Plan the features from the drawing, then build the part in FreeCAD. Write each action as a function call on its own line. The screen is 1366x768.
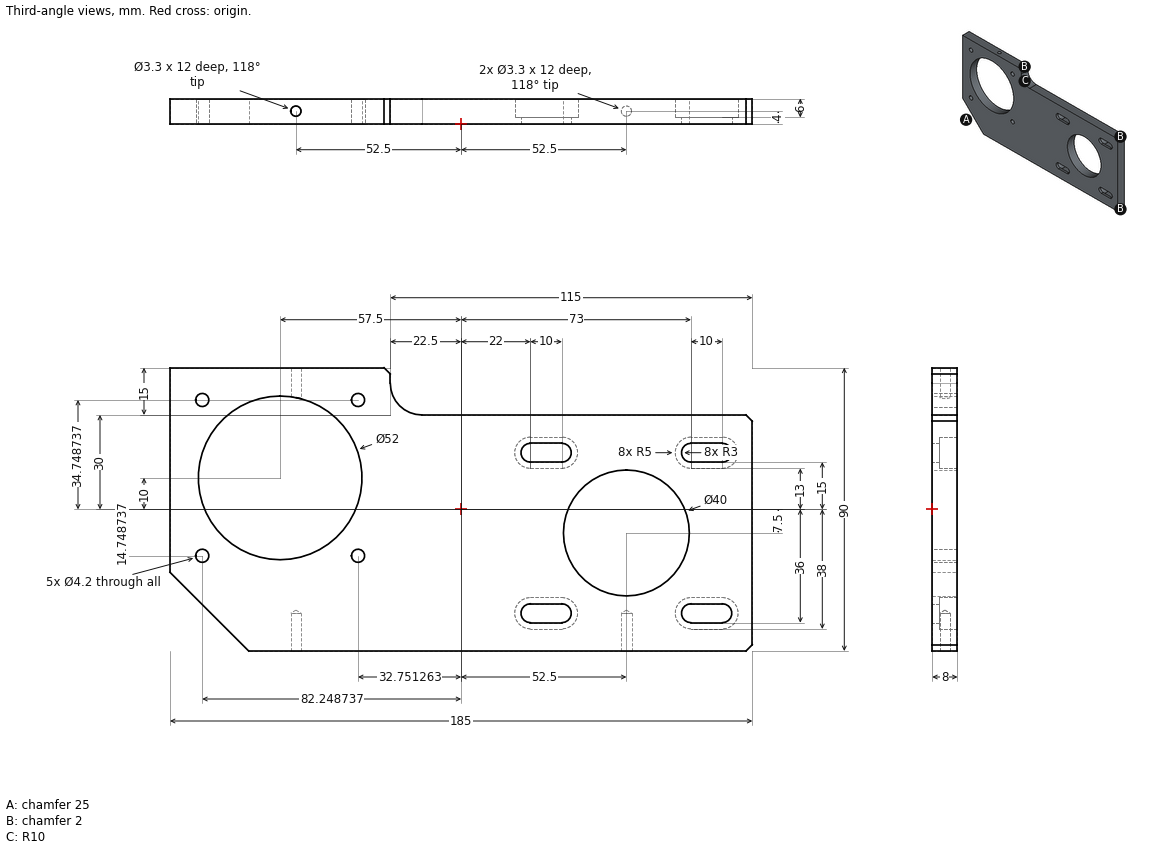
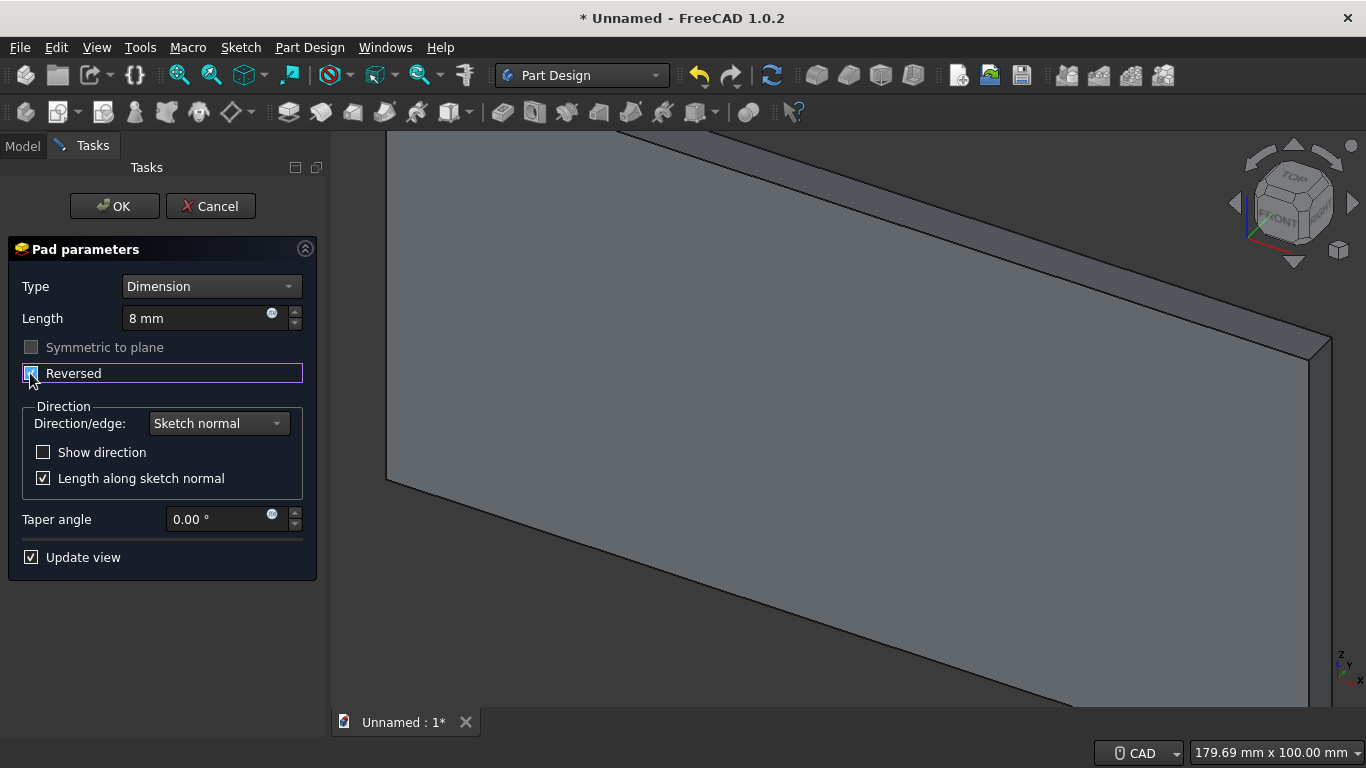
click(115, 206)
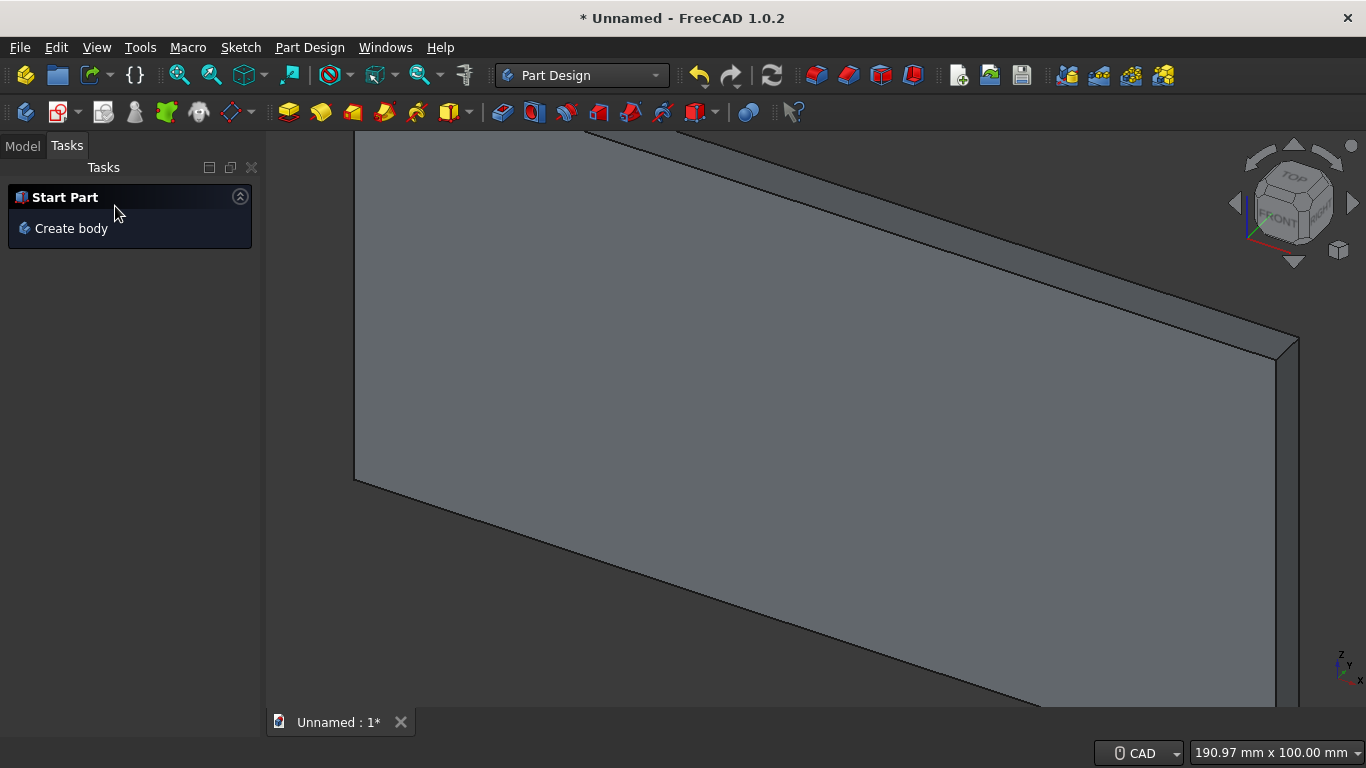
click(180, 76)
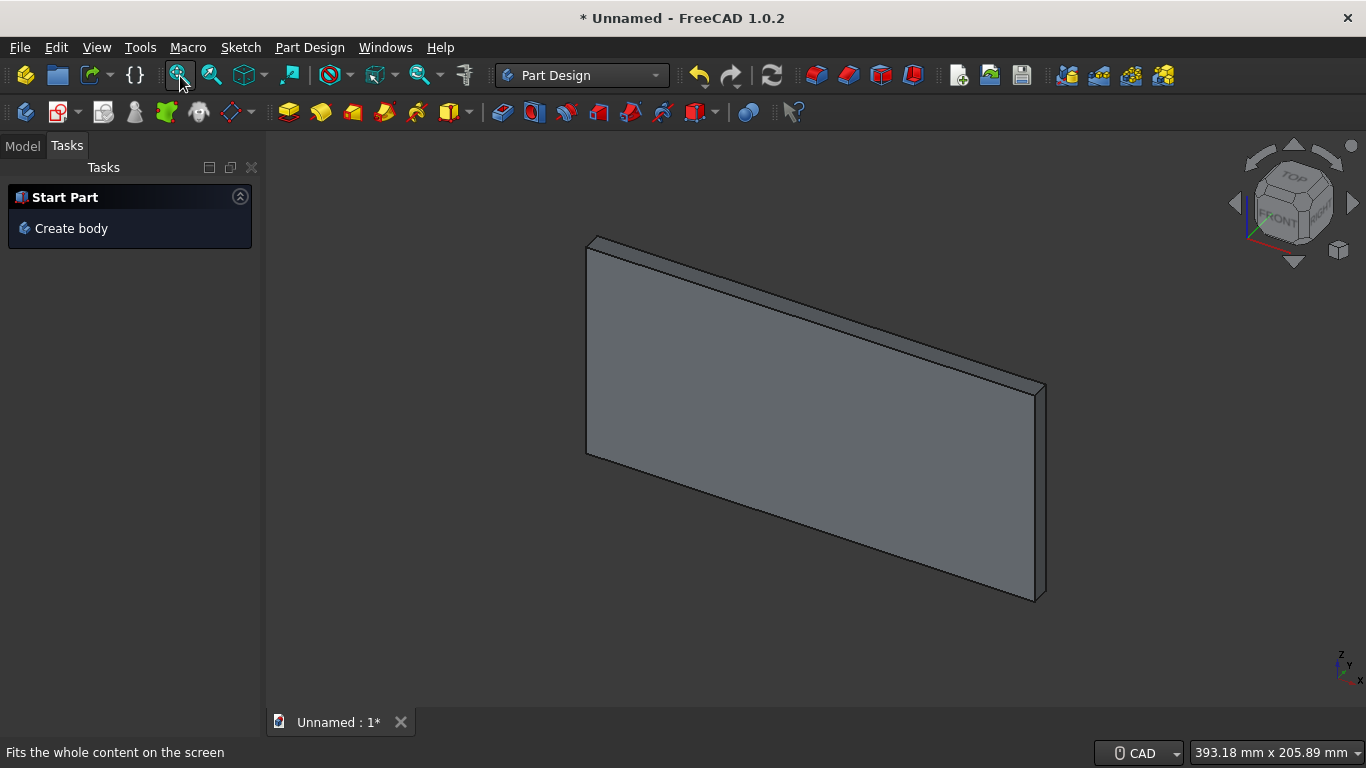
key(4)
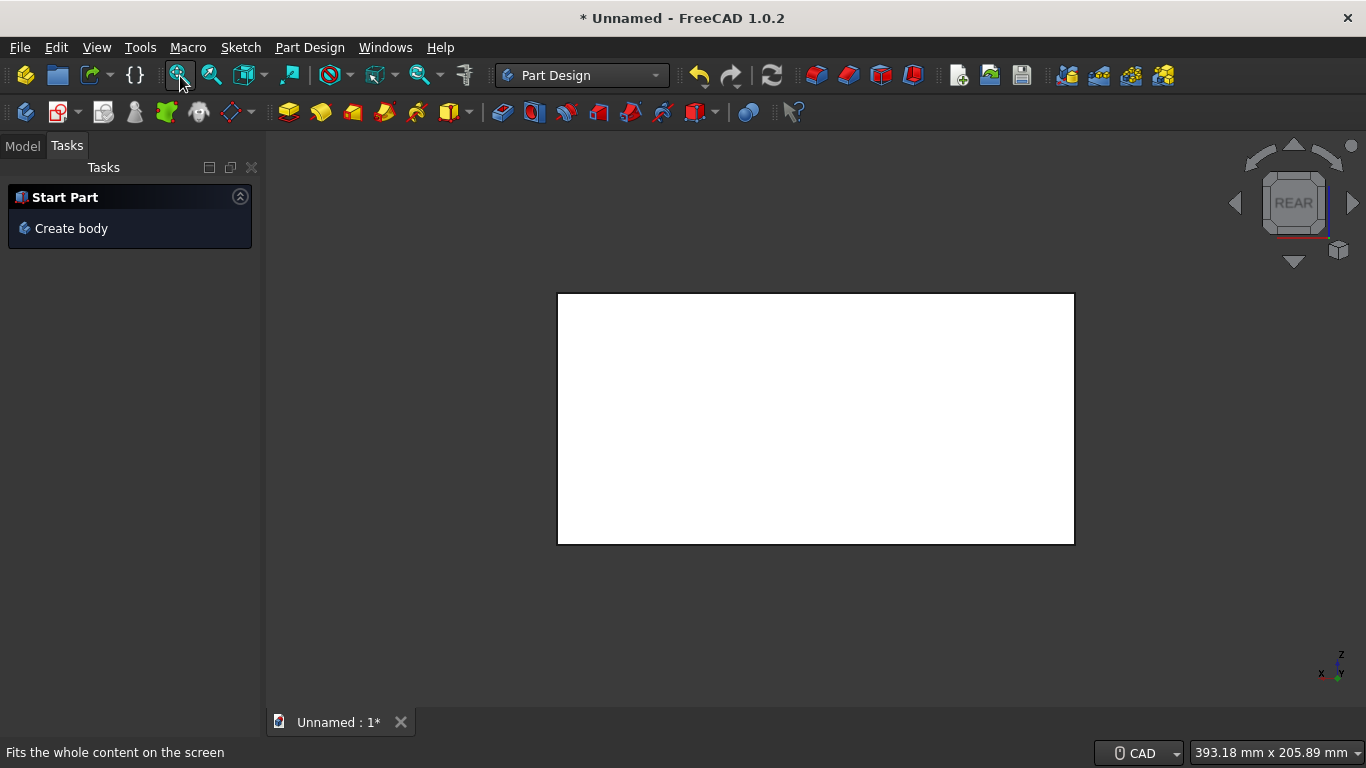
click(742, 418)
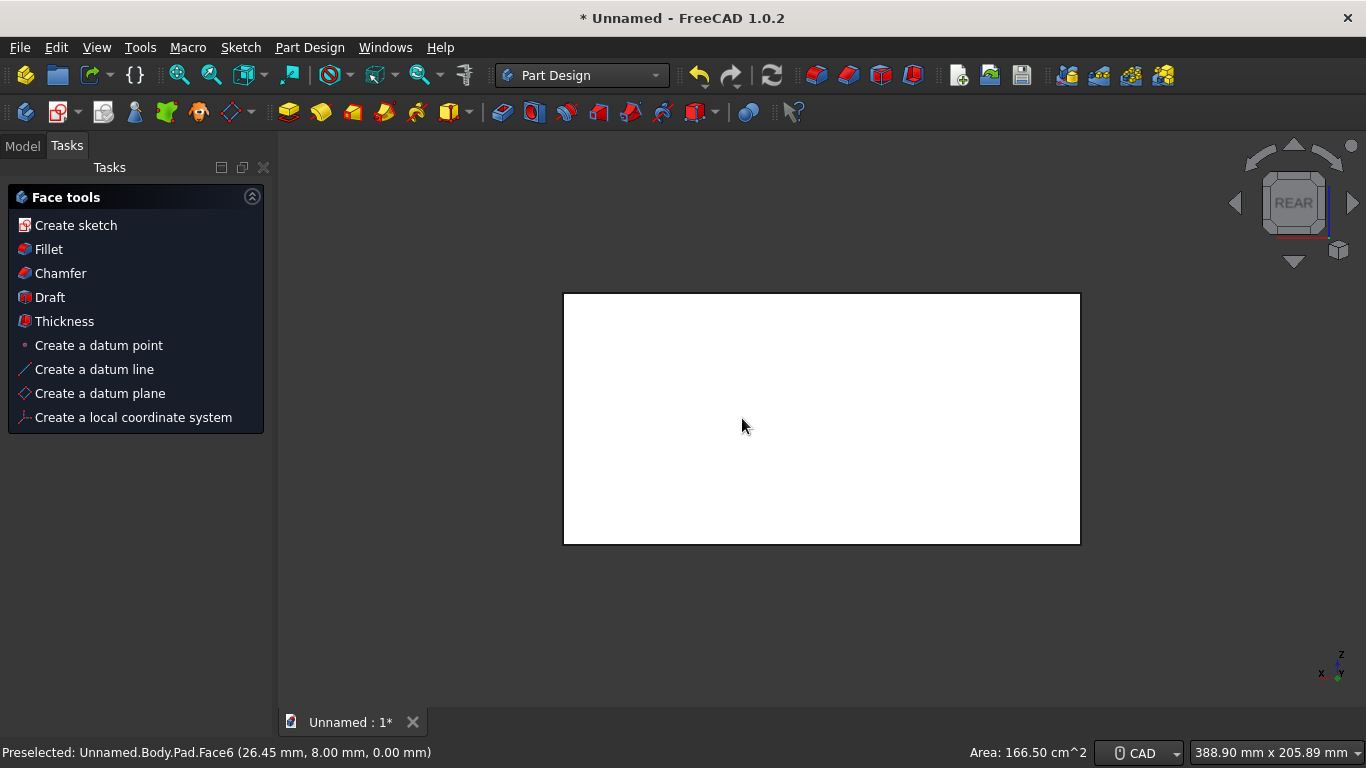
click(58, 112)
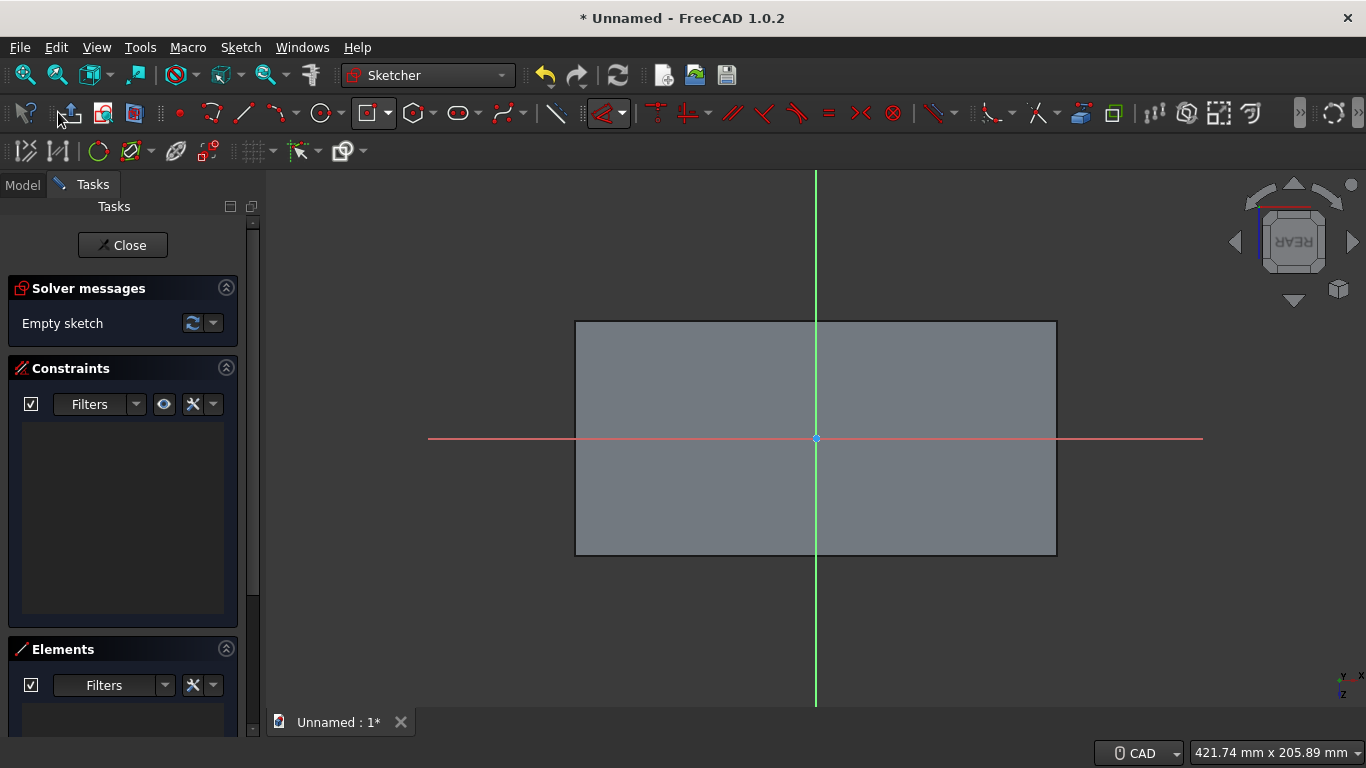
scroll(1038, 545, up, 4)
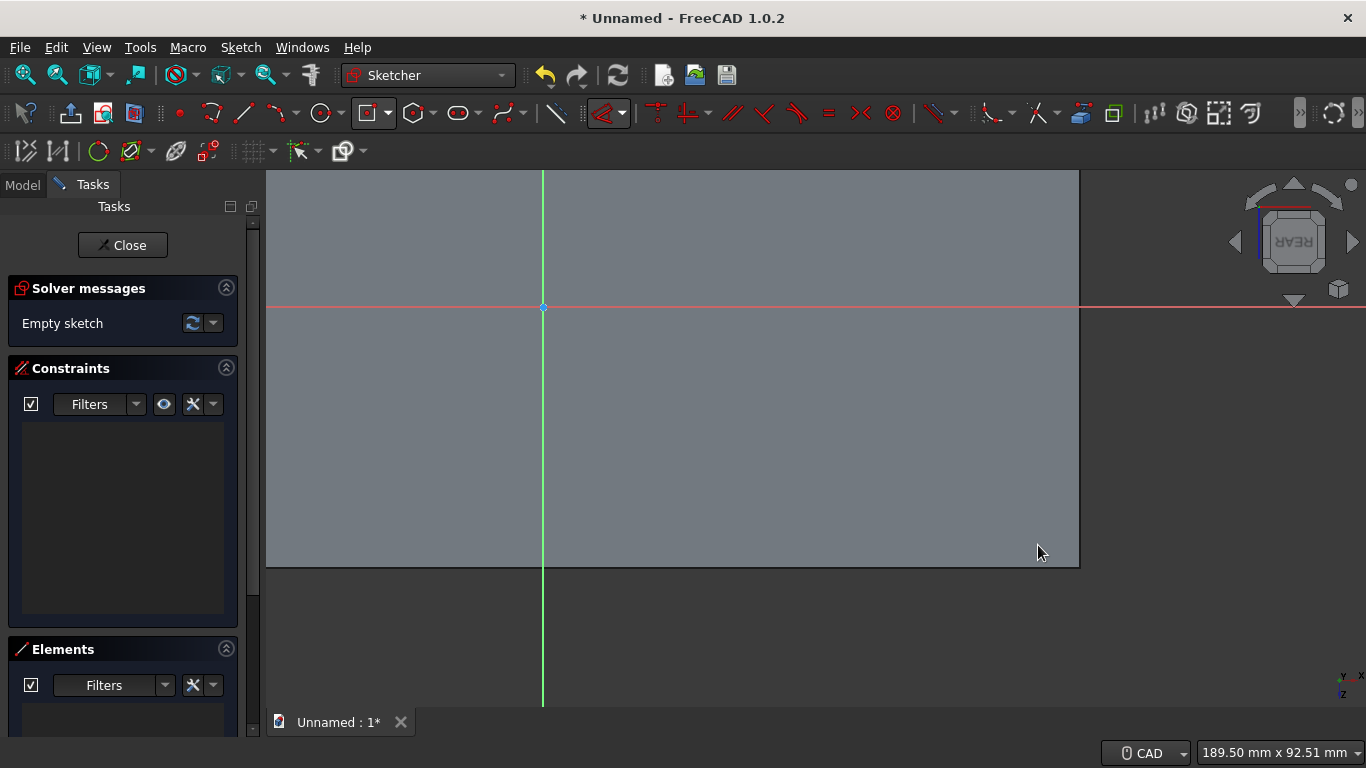
key(g)
key(r)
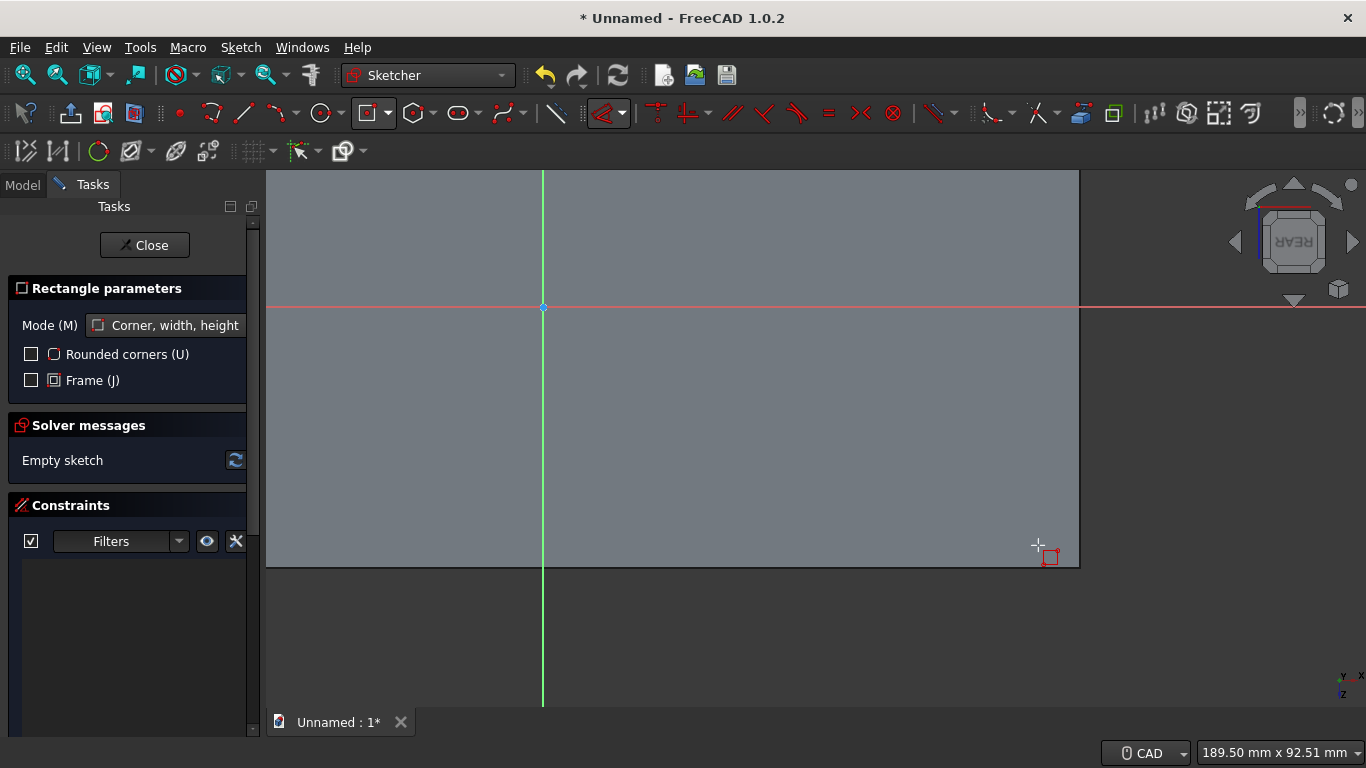
click(412, 481)
click(1080, 568)
key(Escape)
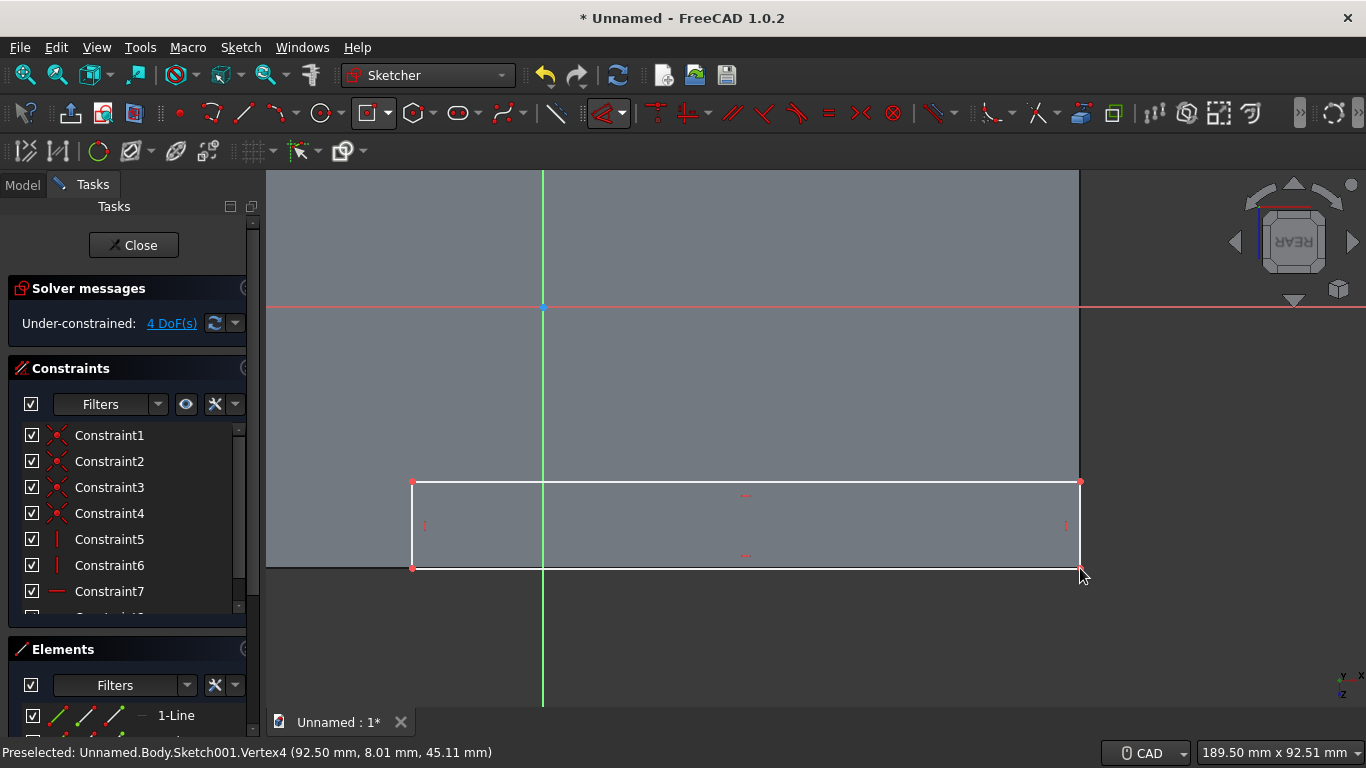
click(412, 508)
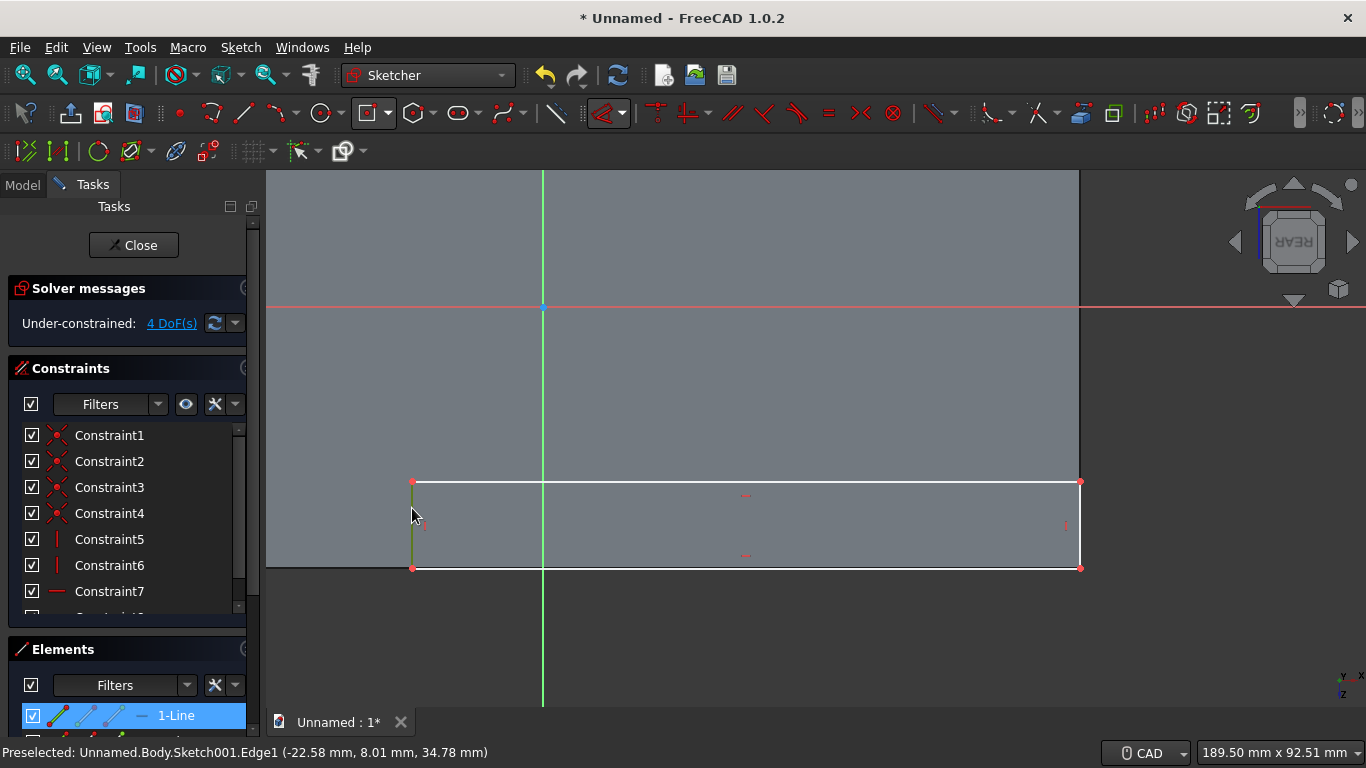
key(i)